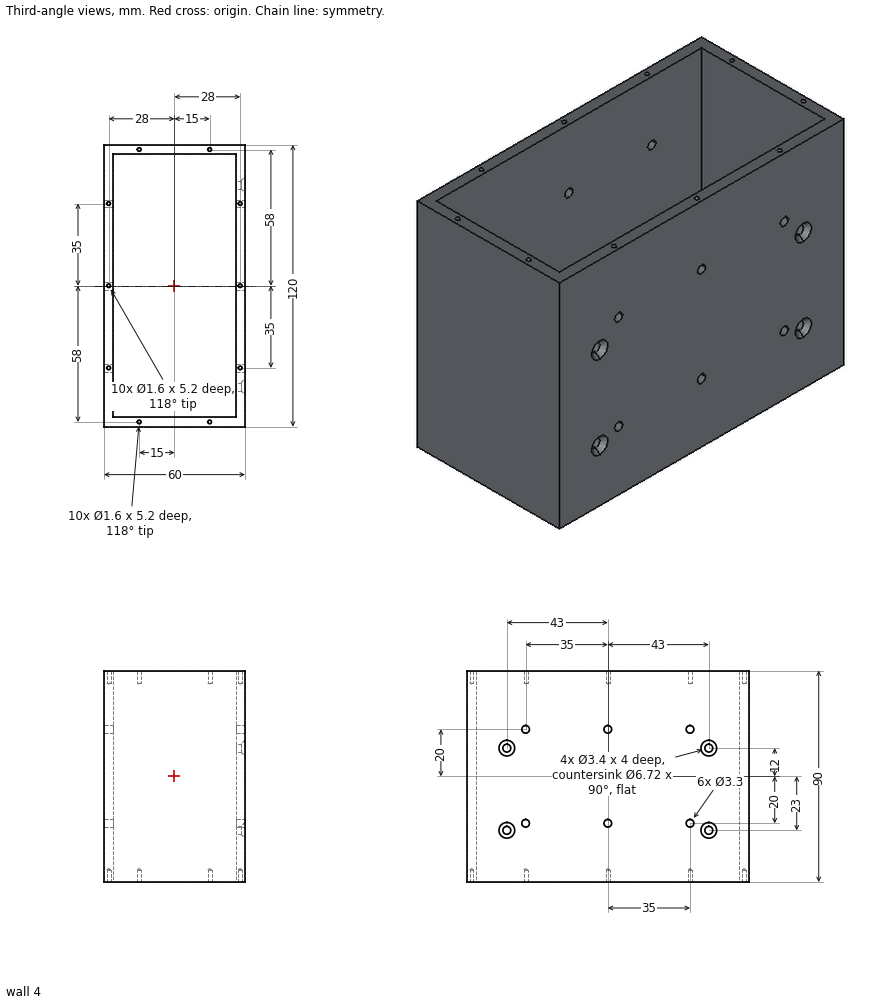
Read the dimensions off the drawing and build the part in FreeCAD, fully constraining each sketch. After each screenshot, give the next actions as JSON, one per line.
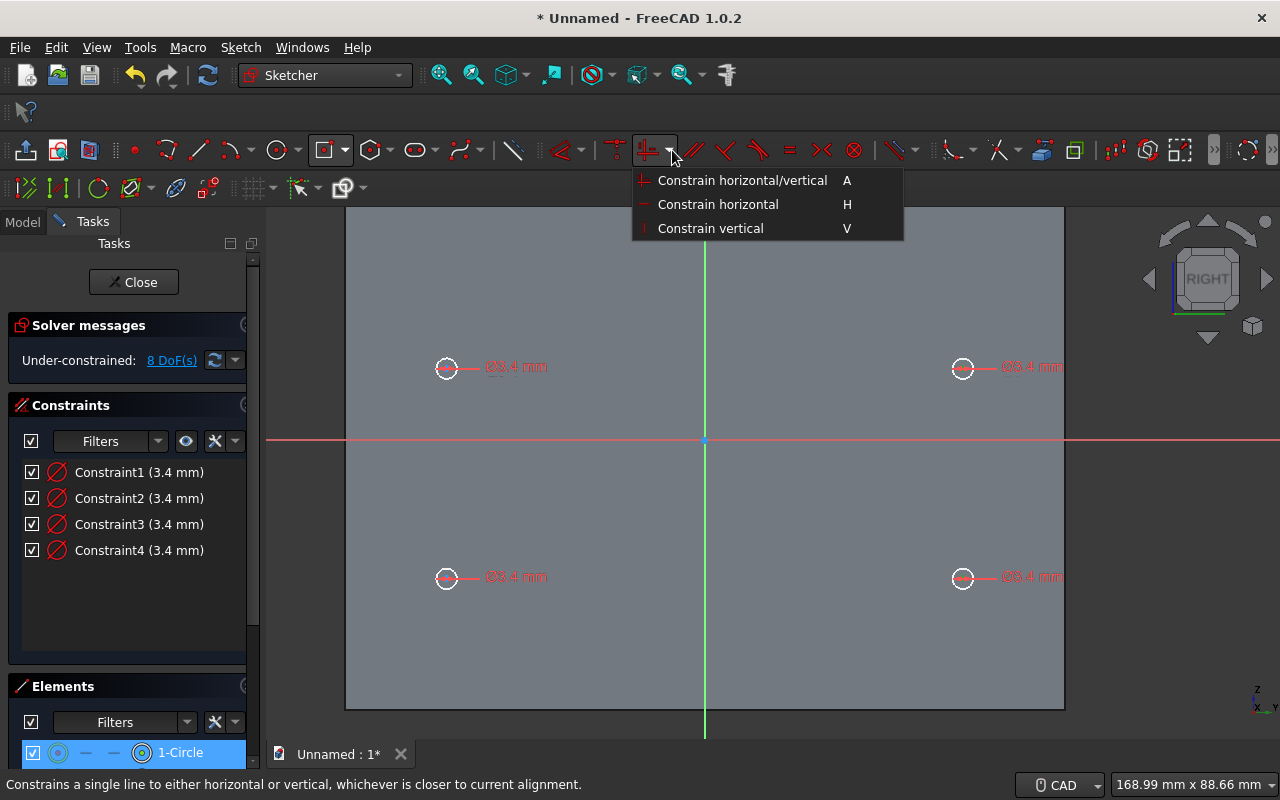
{"action": "left_click", "coordinate": [768, 228]}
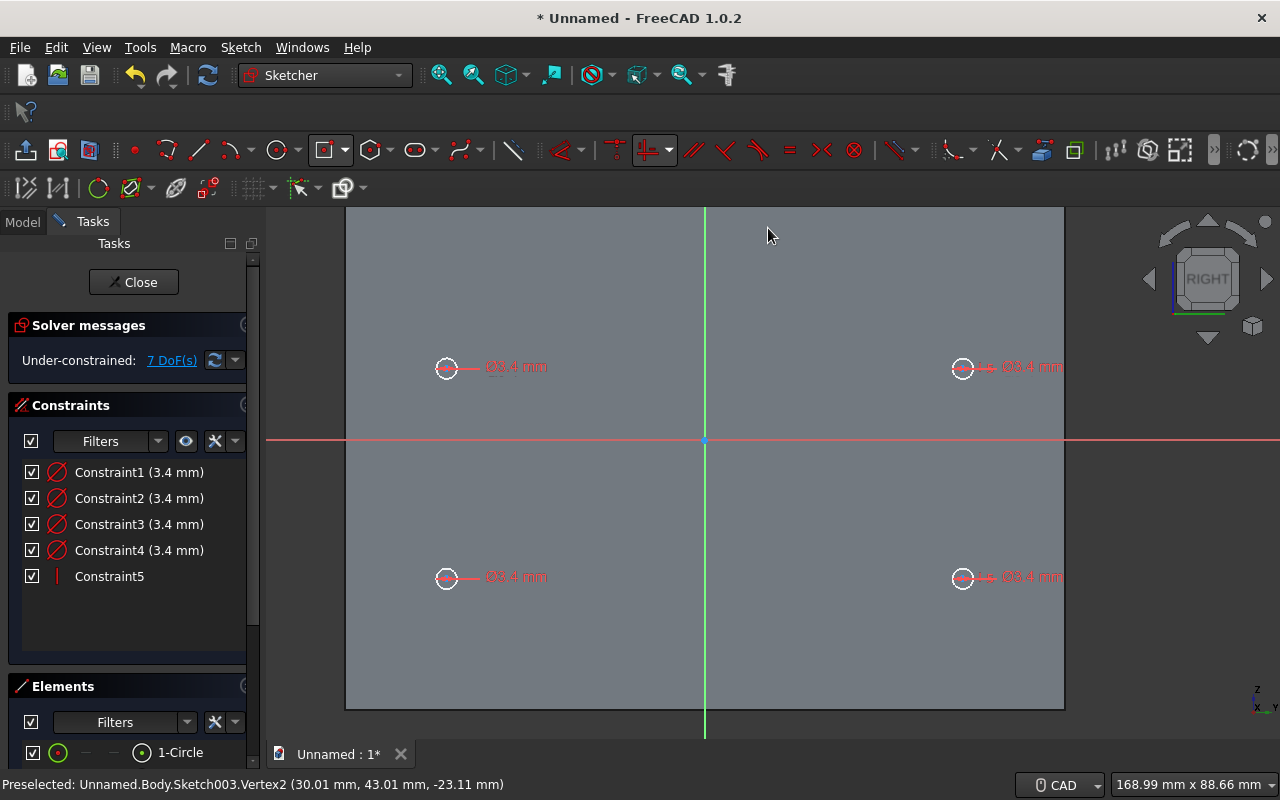
{"action": "left_click", "coordinate": [963, 369]}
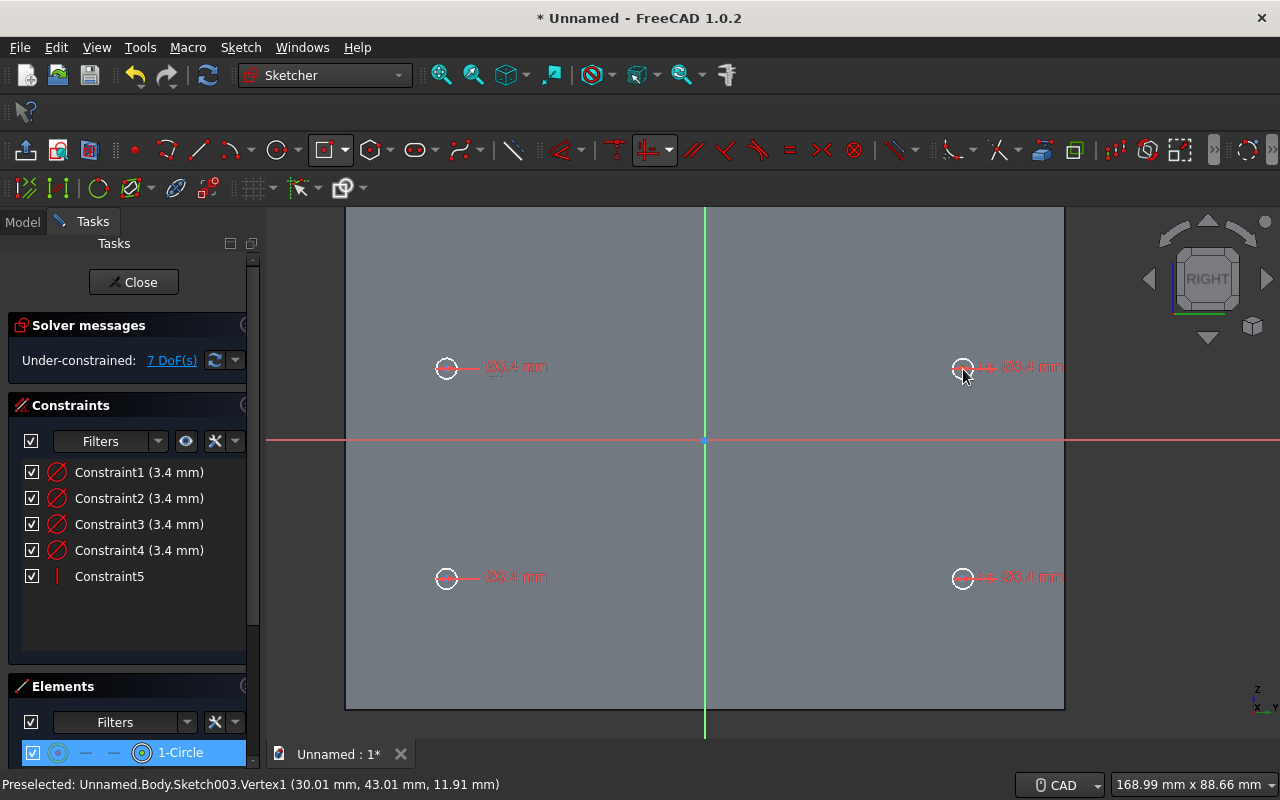
{"action": "left_click", "coordinate": [447, 369]}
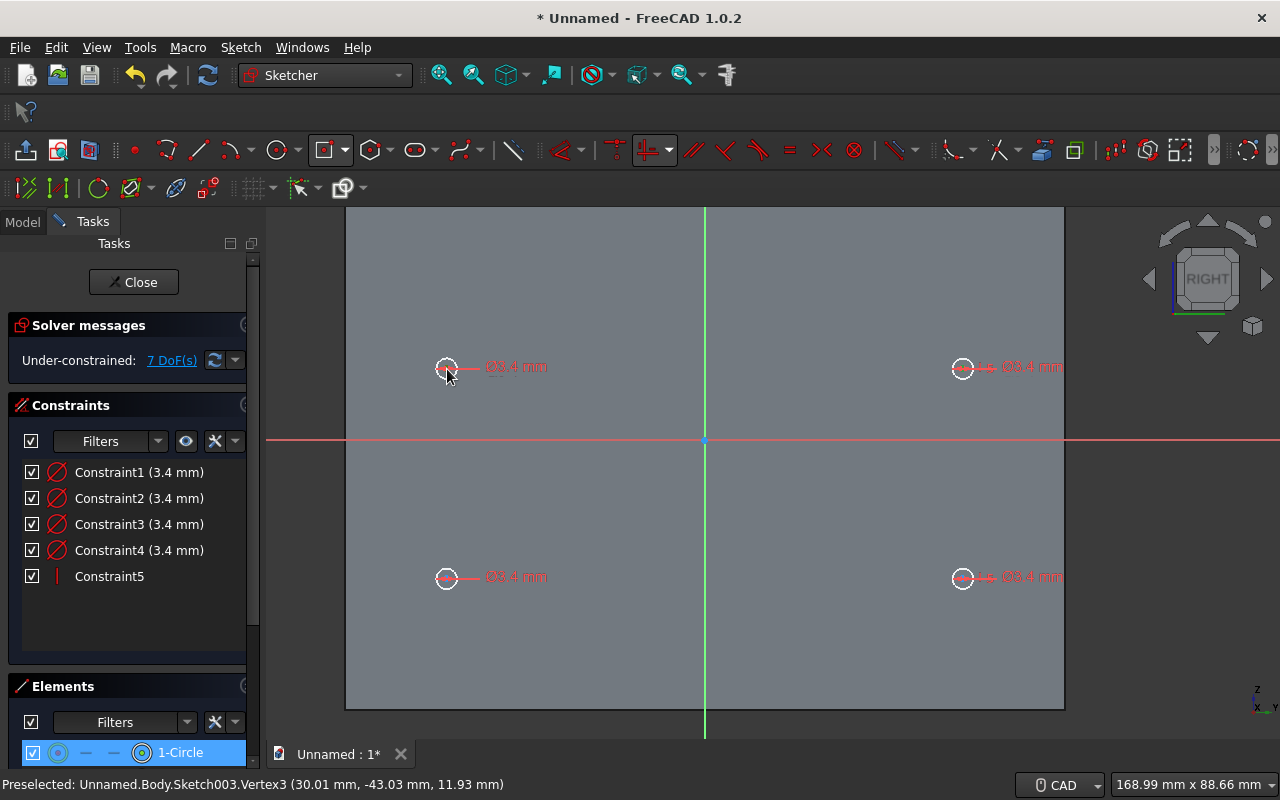
{"action": "left_click", "coordinate": [672, 150]}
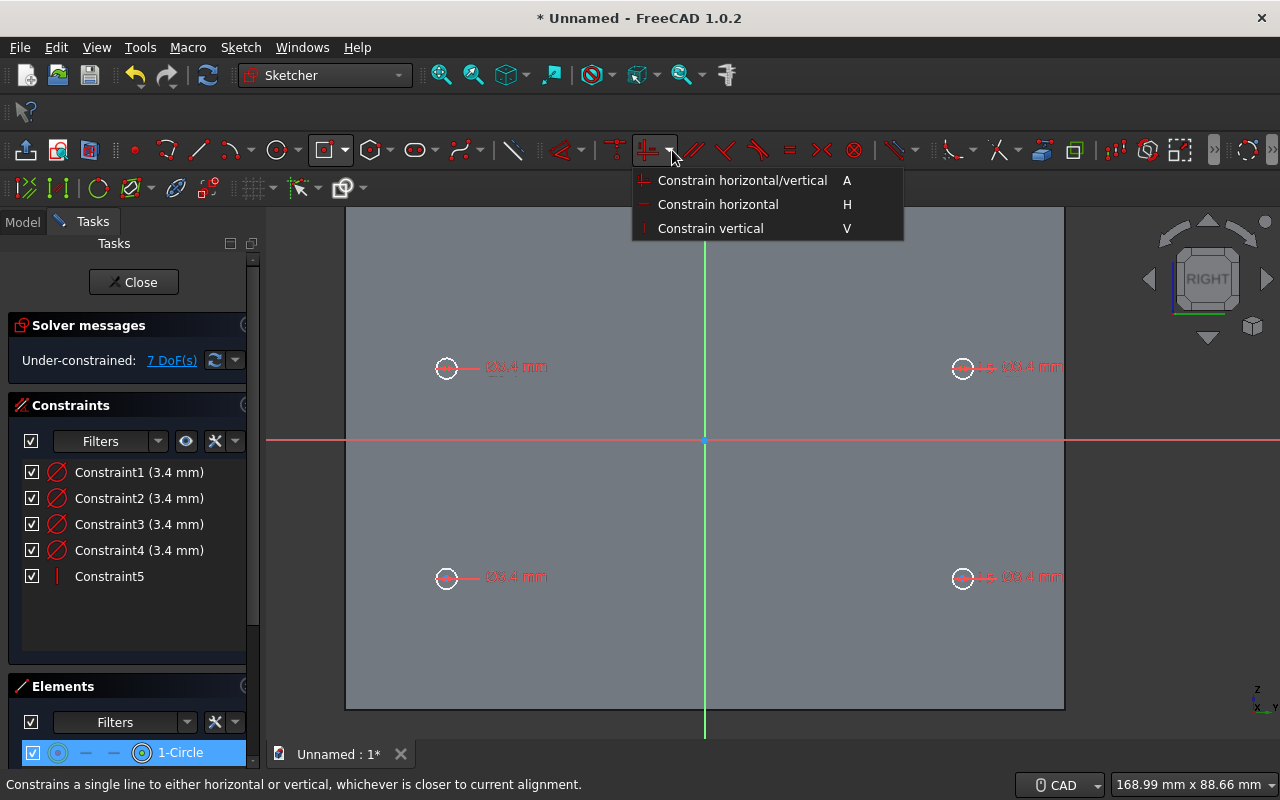
{"action": "left_click", "coordinate": [768, 204]}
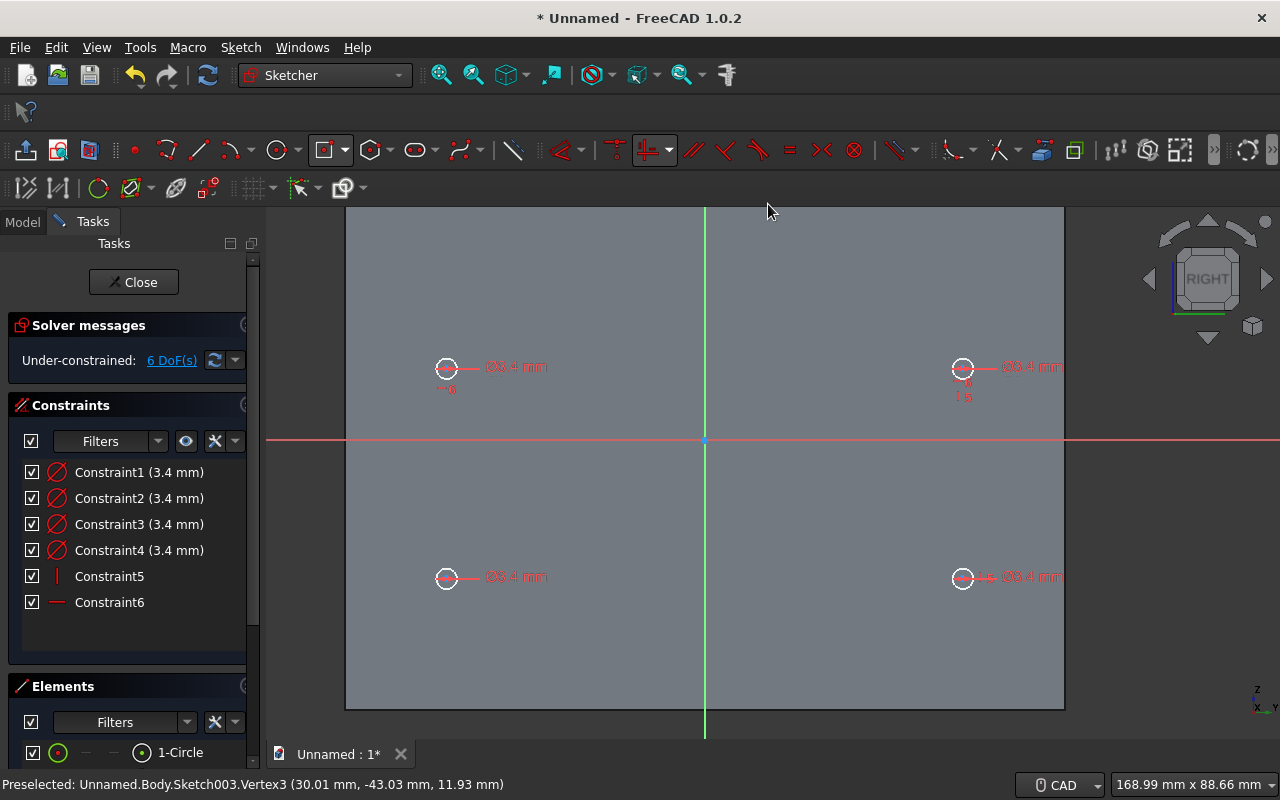
{"action": "left_click", "coordinate": [447, 369]}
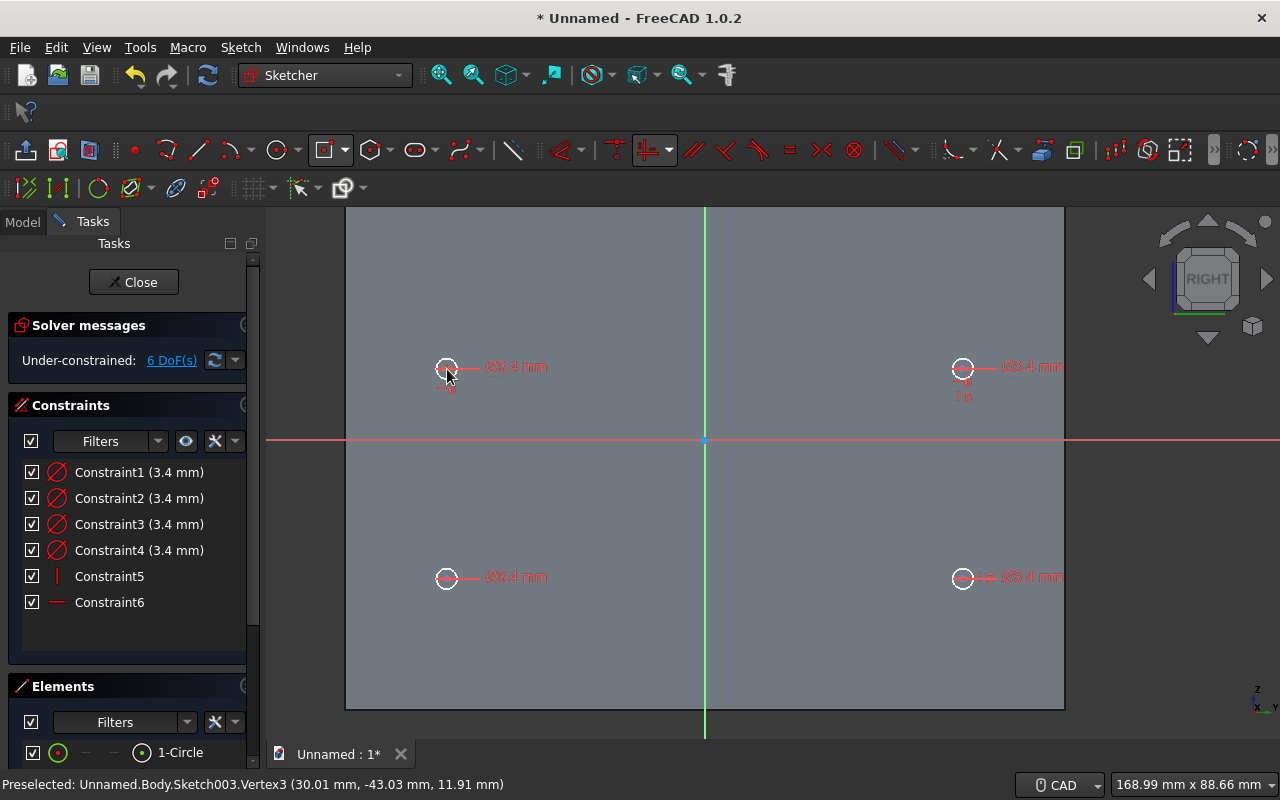
{"action": "left_click", "coordinate": [447, 579]}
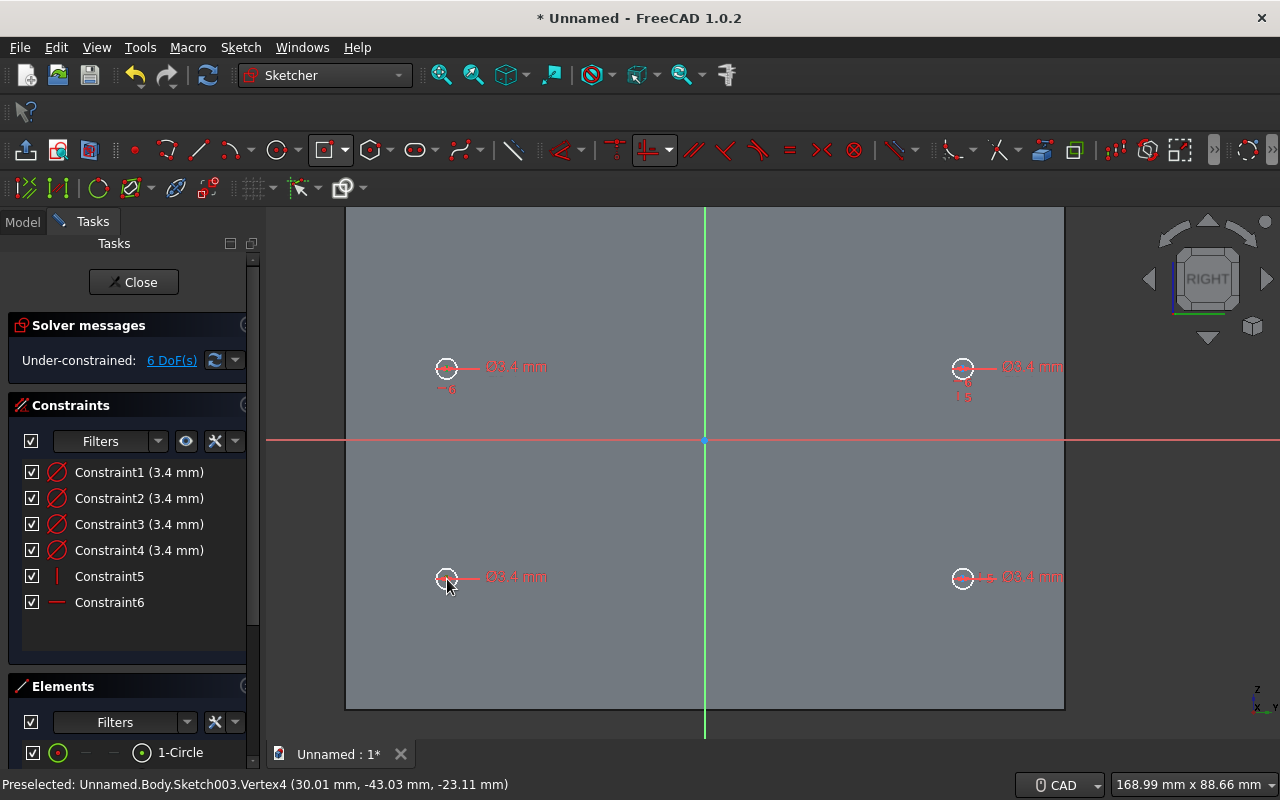
{"action": "key", "text": "v"}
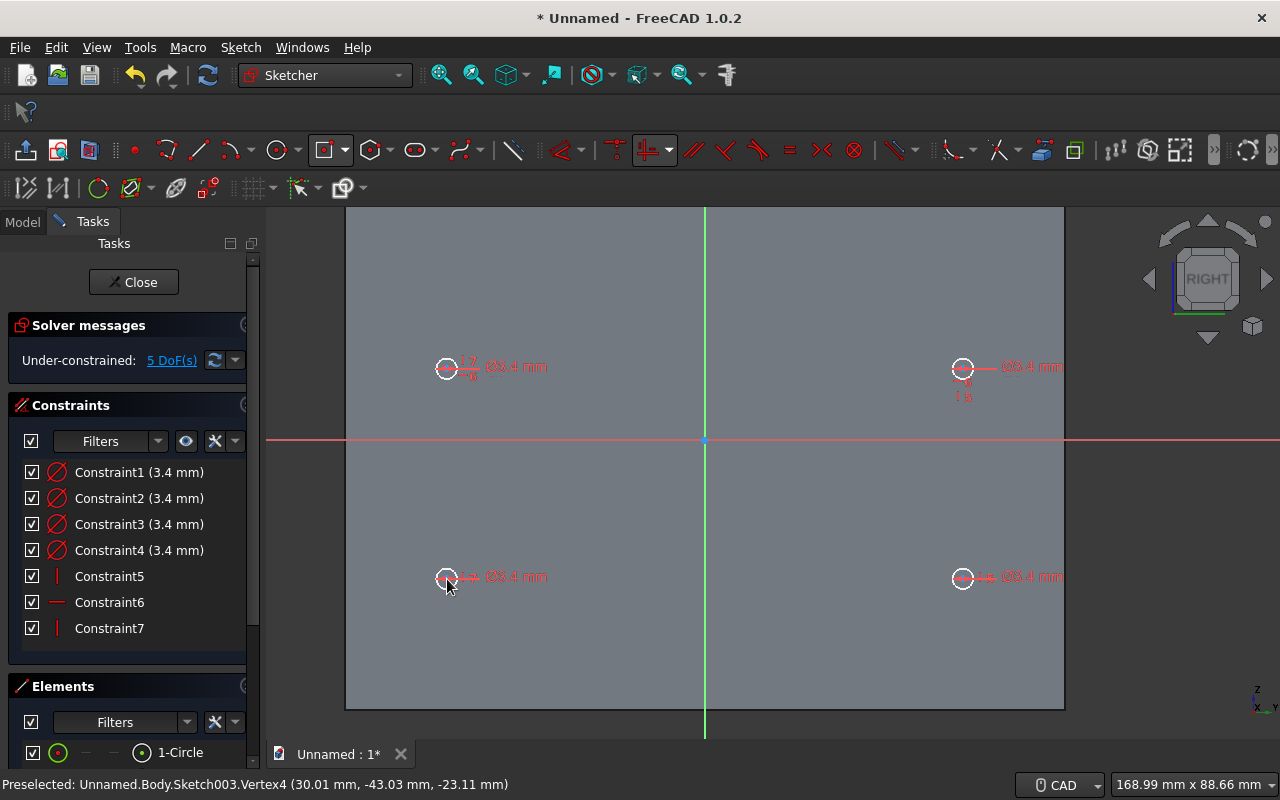
{"action": "left_click", "coordinate": [963, 579]}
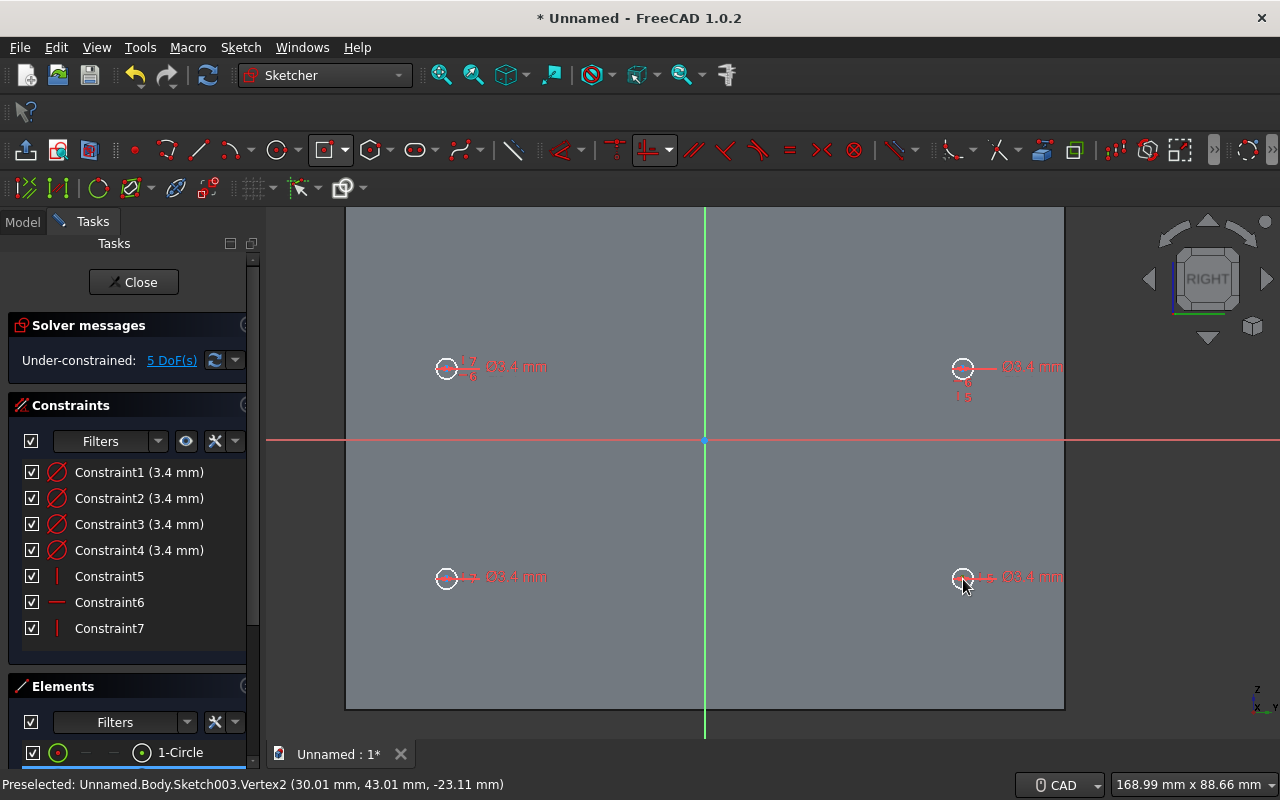
{"action": "left_click", "coordinate": [447, 579]}